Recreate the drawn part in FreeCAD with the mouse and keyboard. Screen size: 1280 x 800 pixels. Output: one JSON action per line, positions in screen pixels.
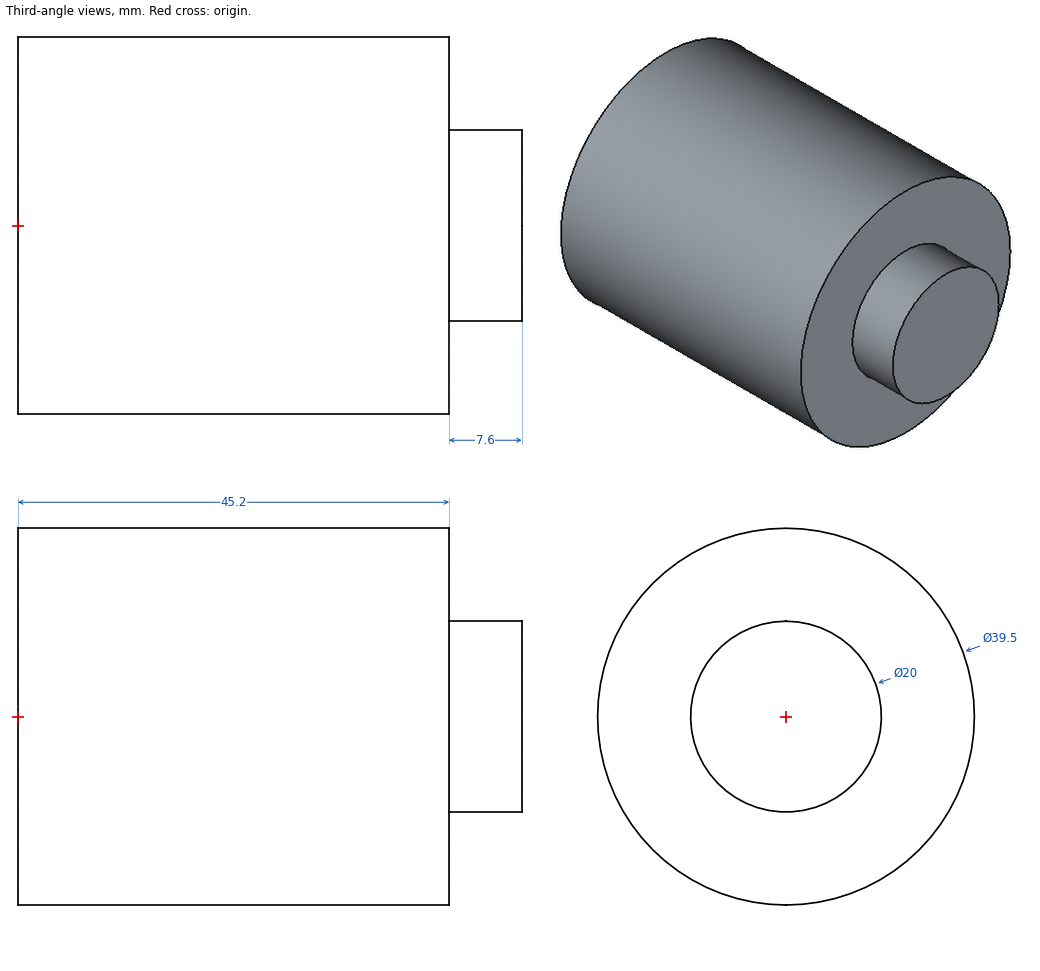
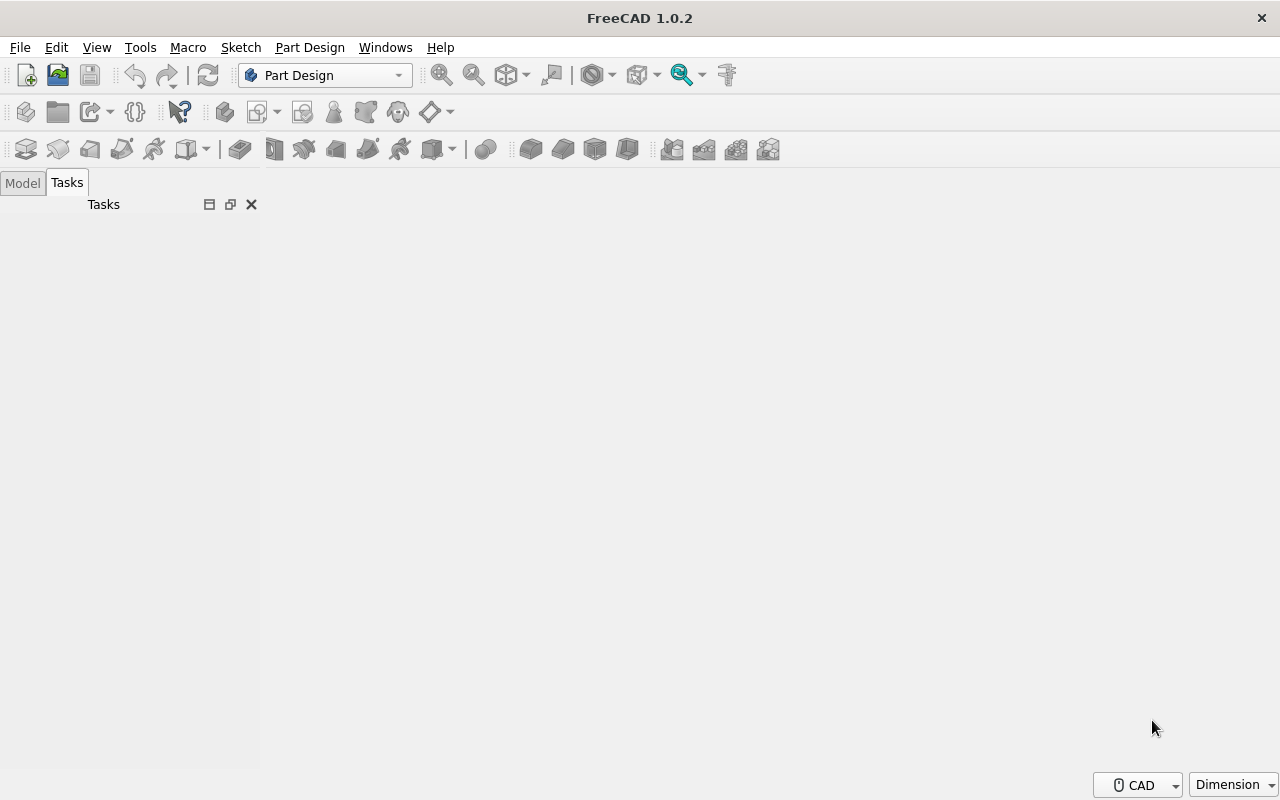
{"action": "left_click", "coordinate": [286, 112]}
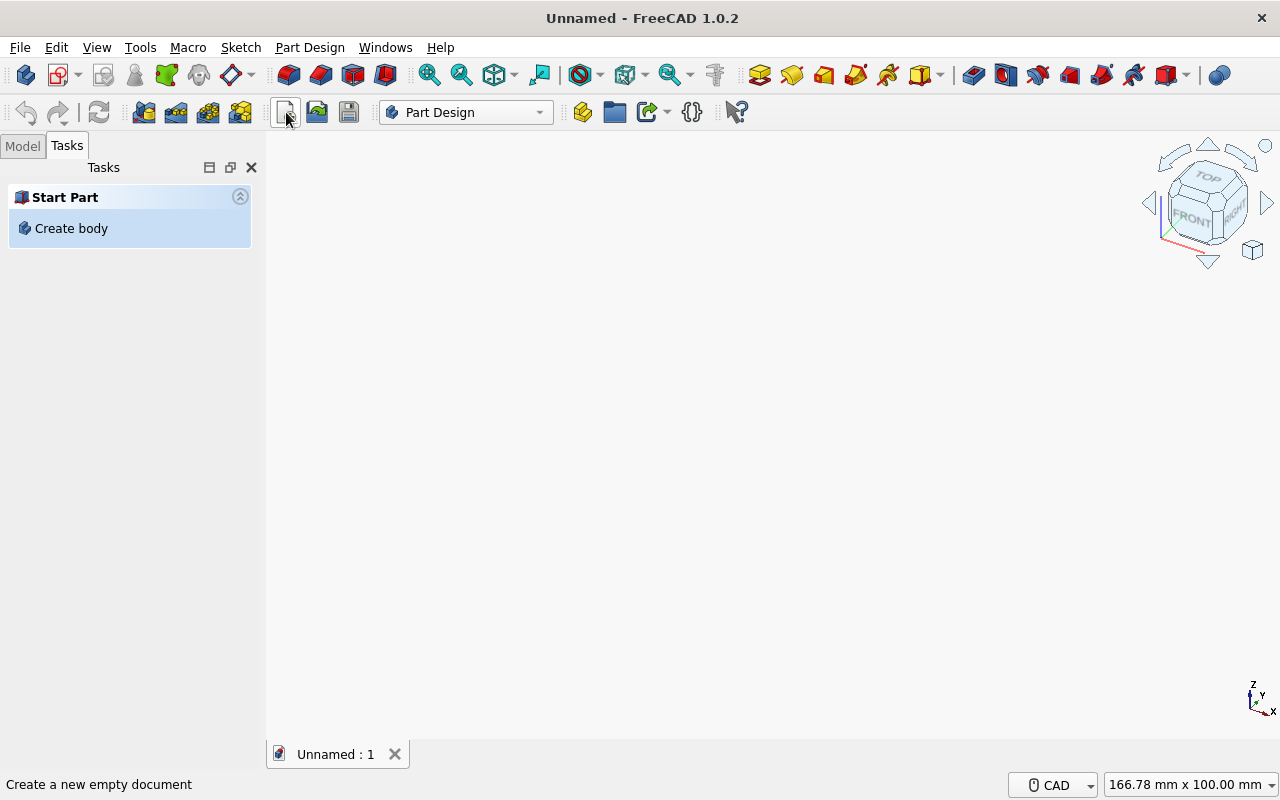
{"action": "left_click", "coordinate": [58, 76]}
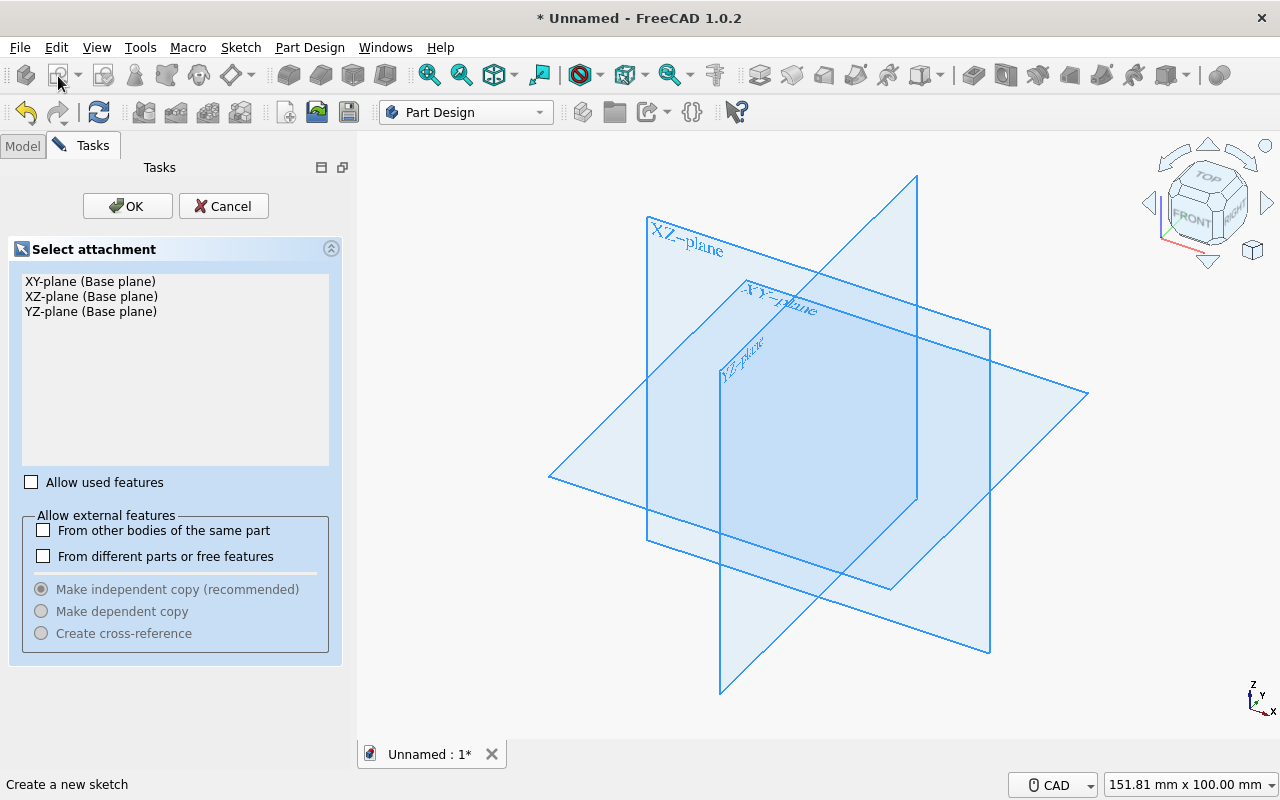
{"action": "left_click", "coordinate": [82, 312]}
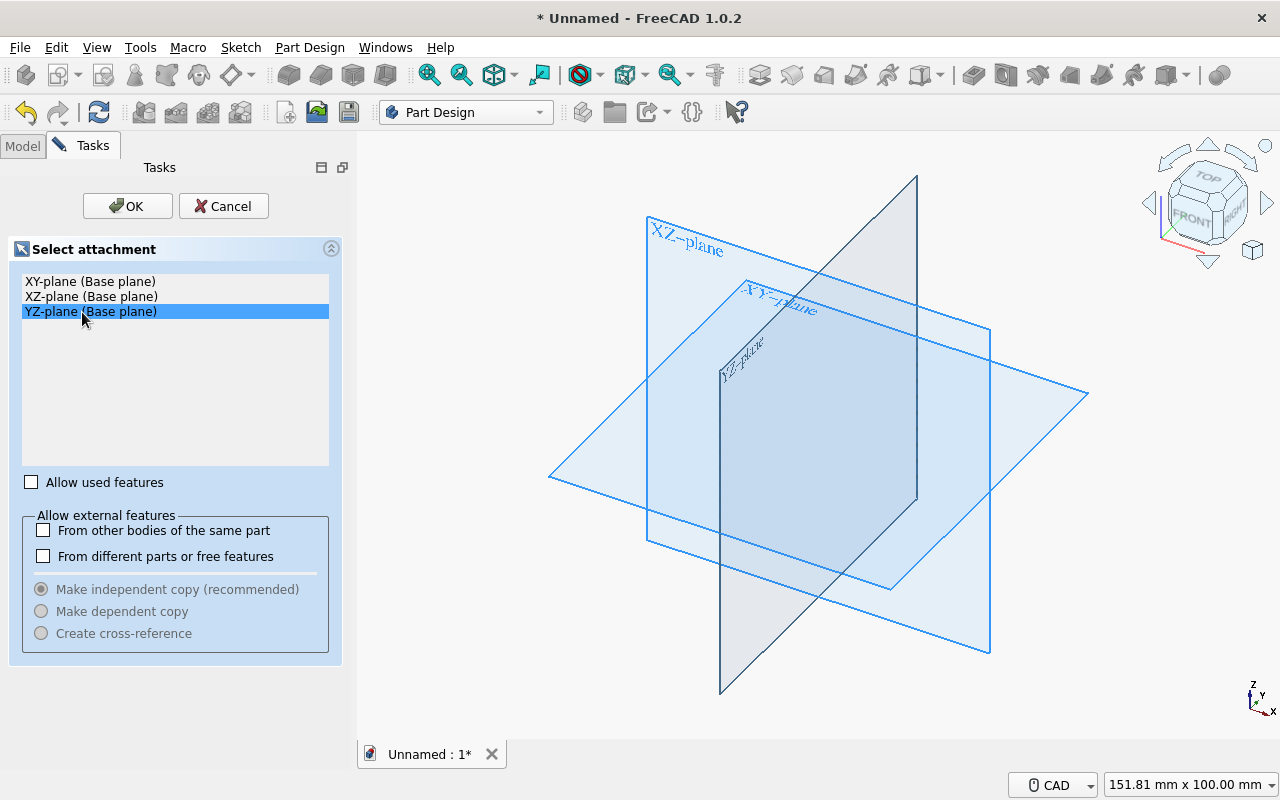
{"action": "left_click", "coordinate": [128, 206]}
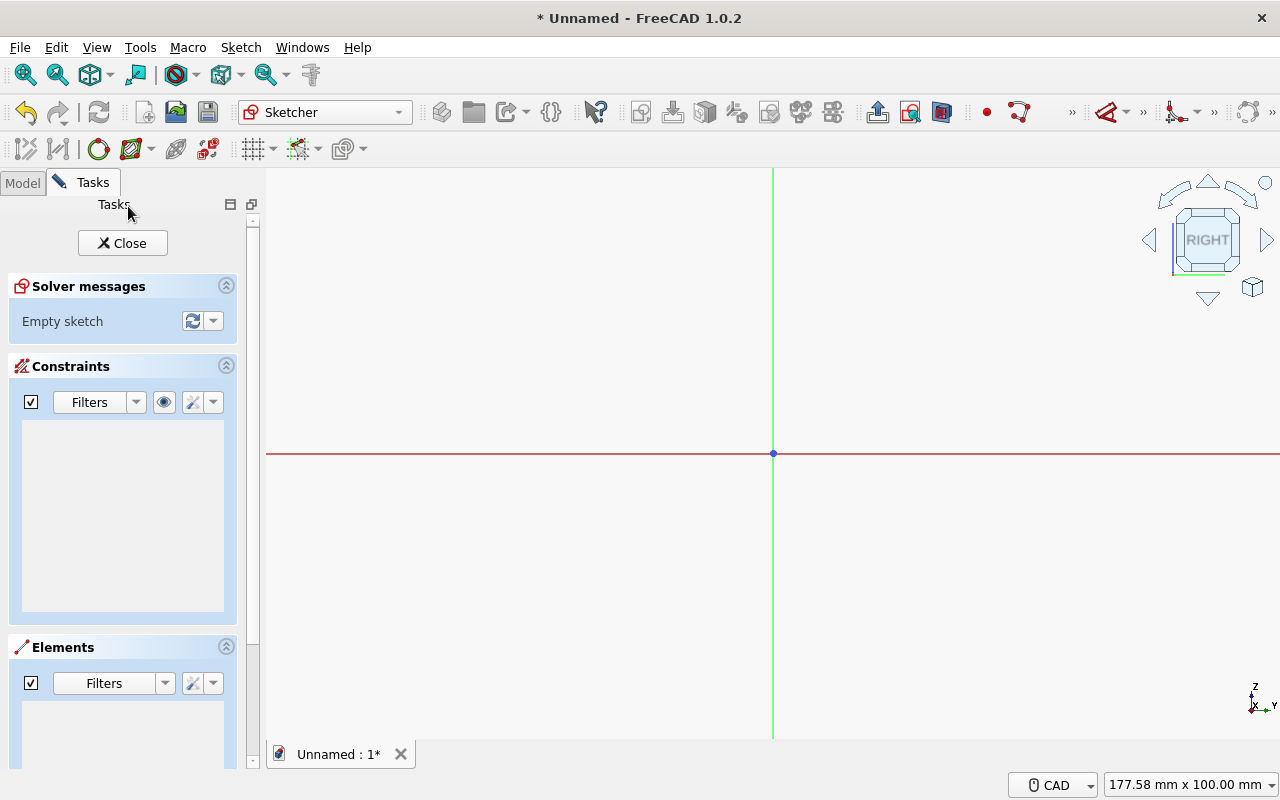
{"action": "scroll", "coordinate": [912, 454], "scroll_direction": "up", "scroll_amount": 2}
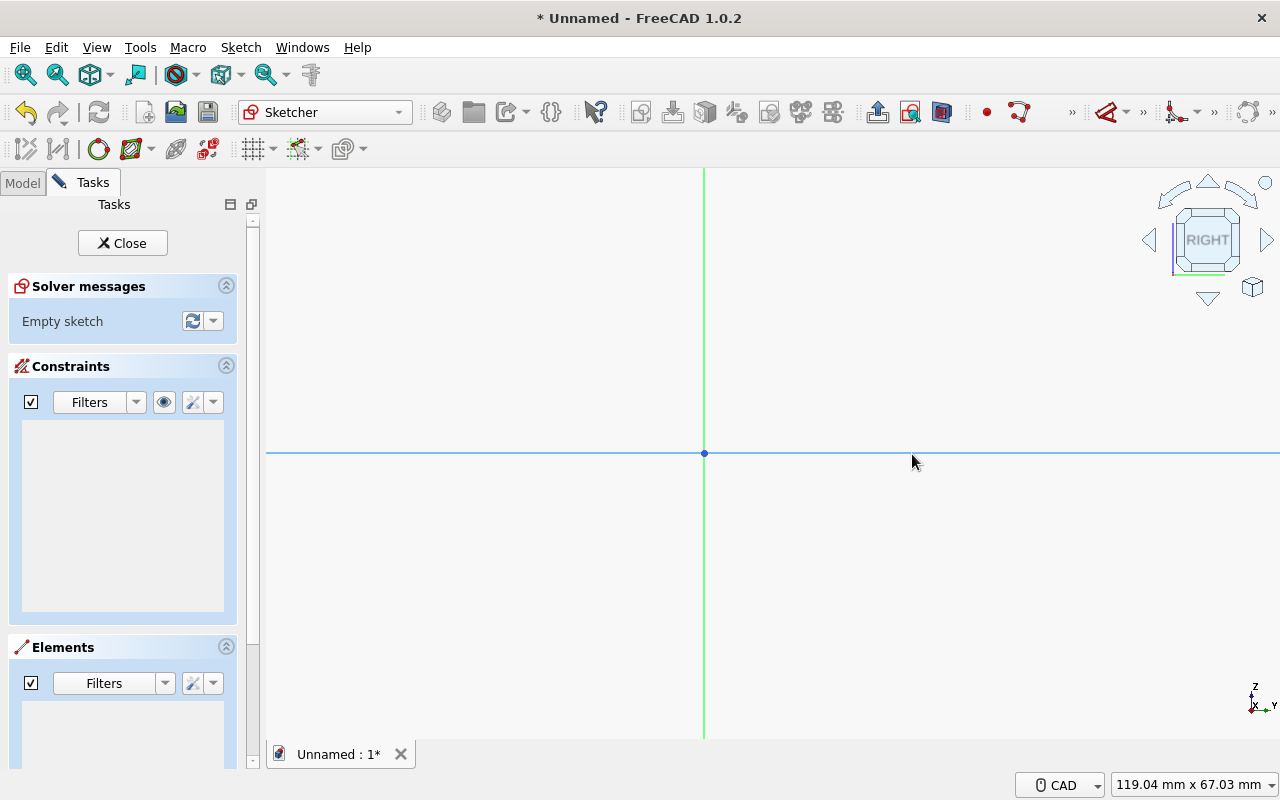
{"action": "key", "text": "g c"}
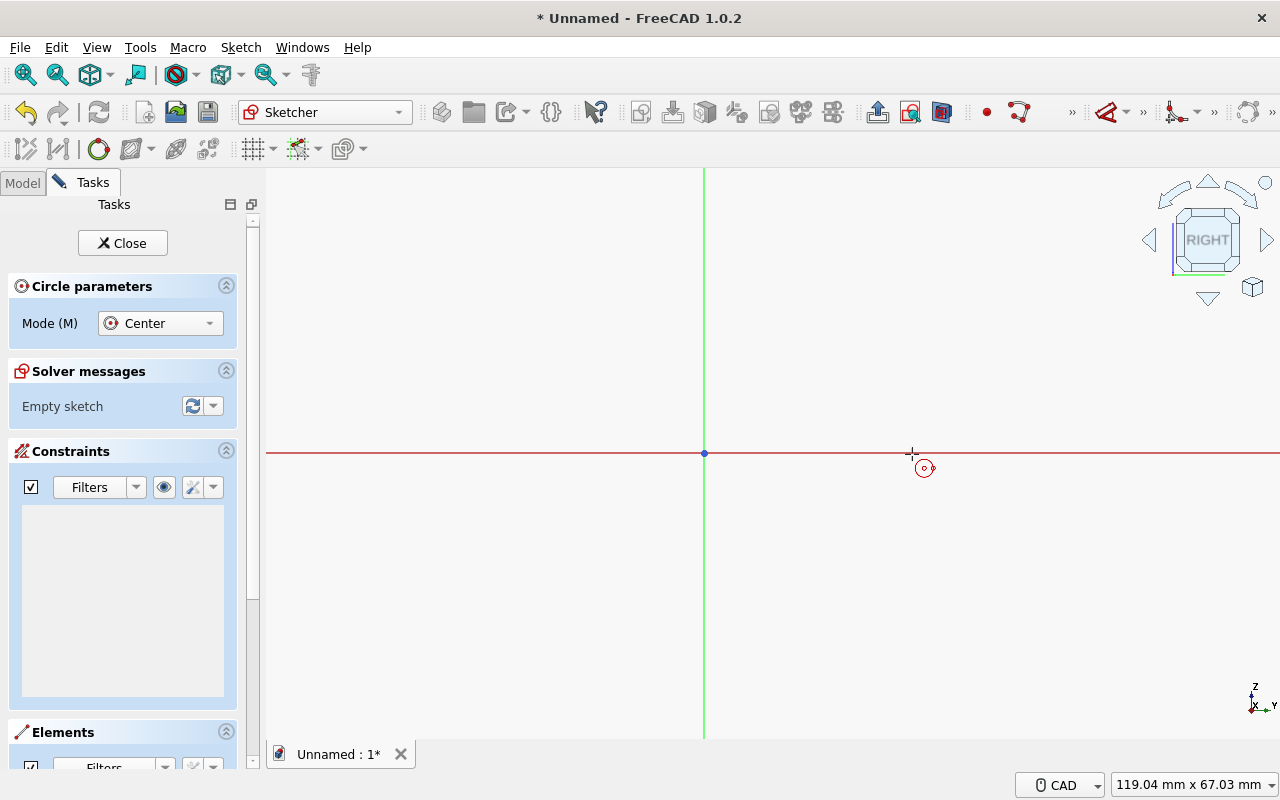
{"action": "left_click", "coordinate": [704, 453]}
{"action": "left_click", "coordinate": [823, 334]}
{"action": "key", "text": "Escape"}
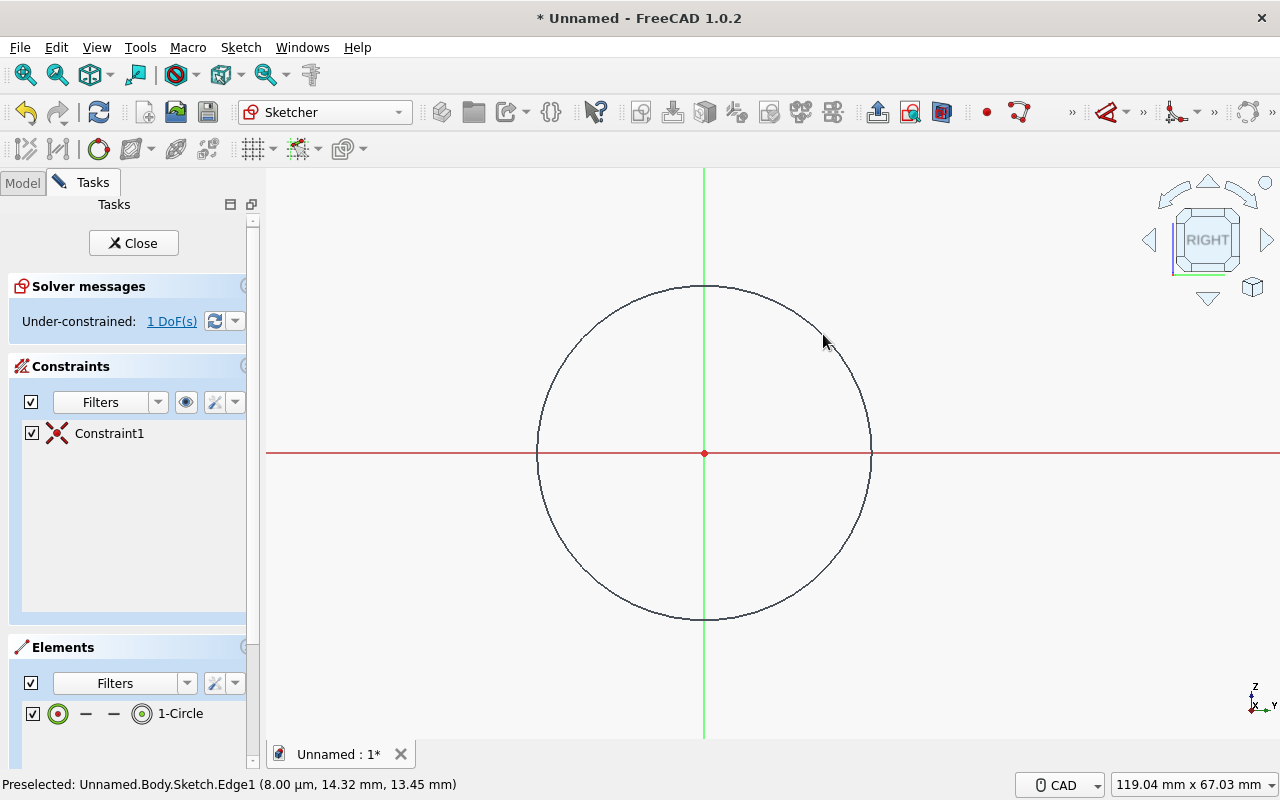
{"action": "left_click", "coordinate": [1106, 112]}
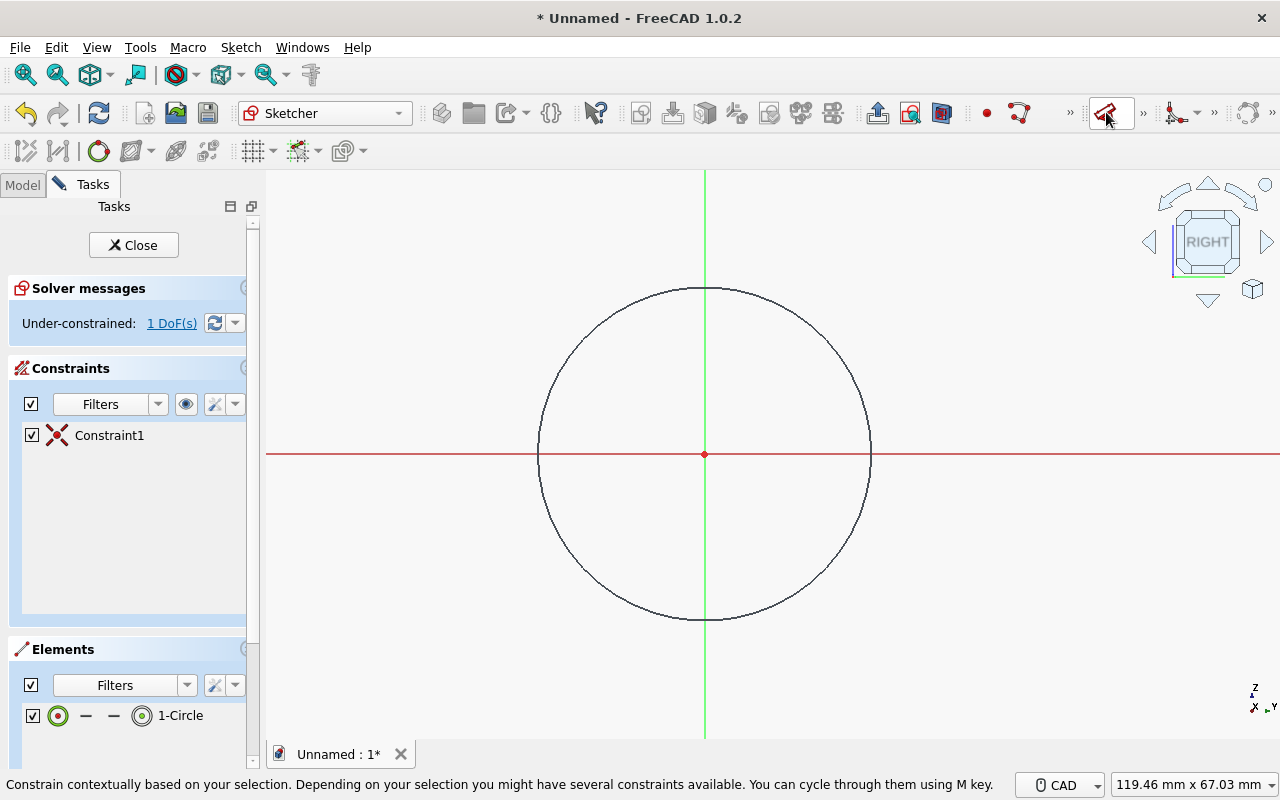
{"action": "left_click", "coordinate": [822, 336]}
{"action": "left_click", "coordinate": [845, 313]}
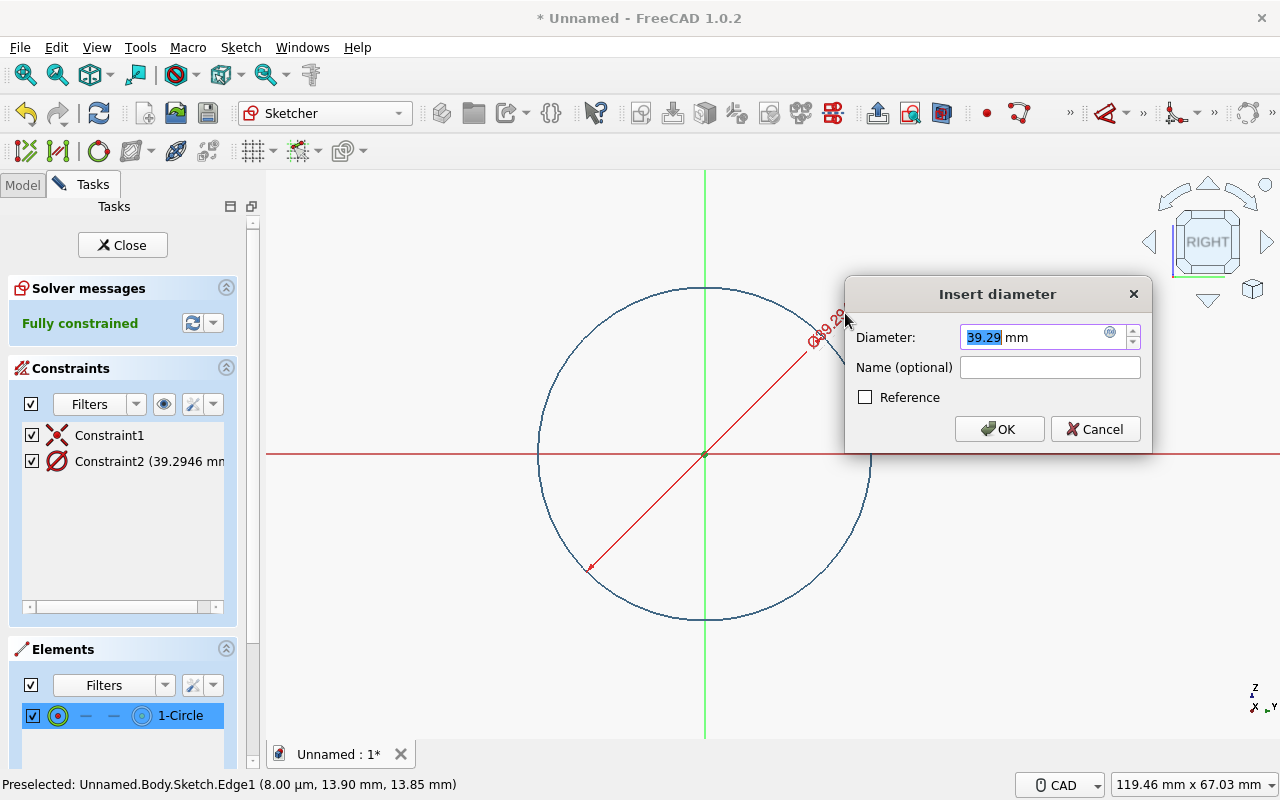
{"action": "type", "text": "39.5"}
{"action": "key", "text": "Return"}
{"action": "key", "text": "Escape"}